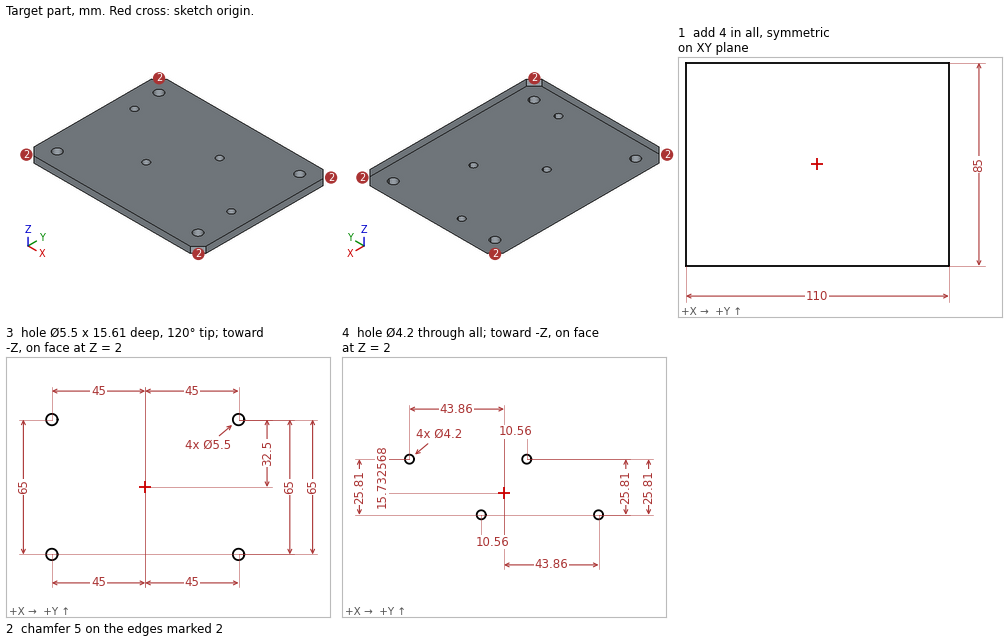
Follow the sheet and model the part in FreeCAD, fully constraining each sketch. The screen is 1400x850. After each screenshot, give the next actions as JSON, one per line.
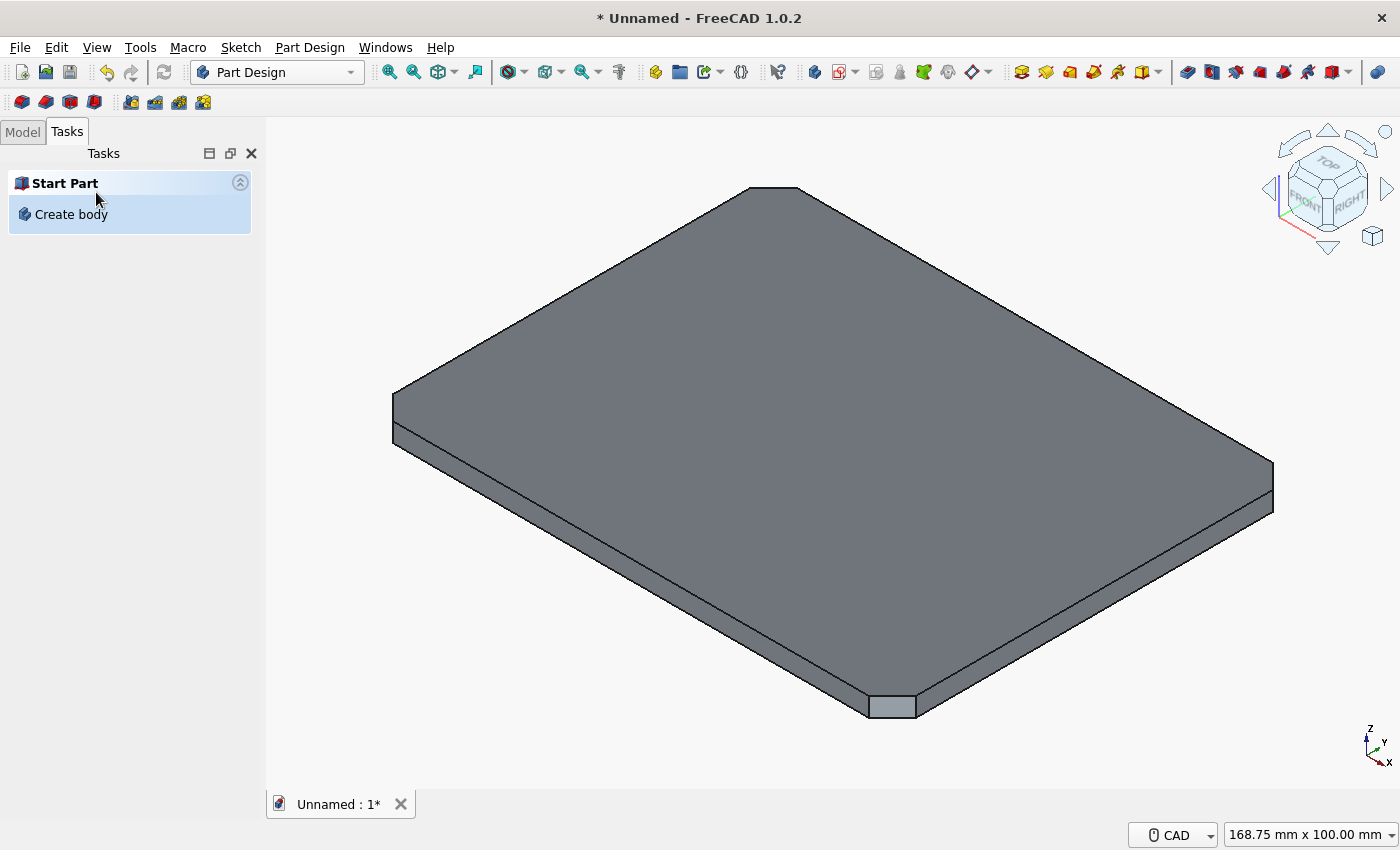
{"action": "left_click", "coordinate": [833, 441]}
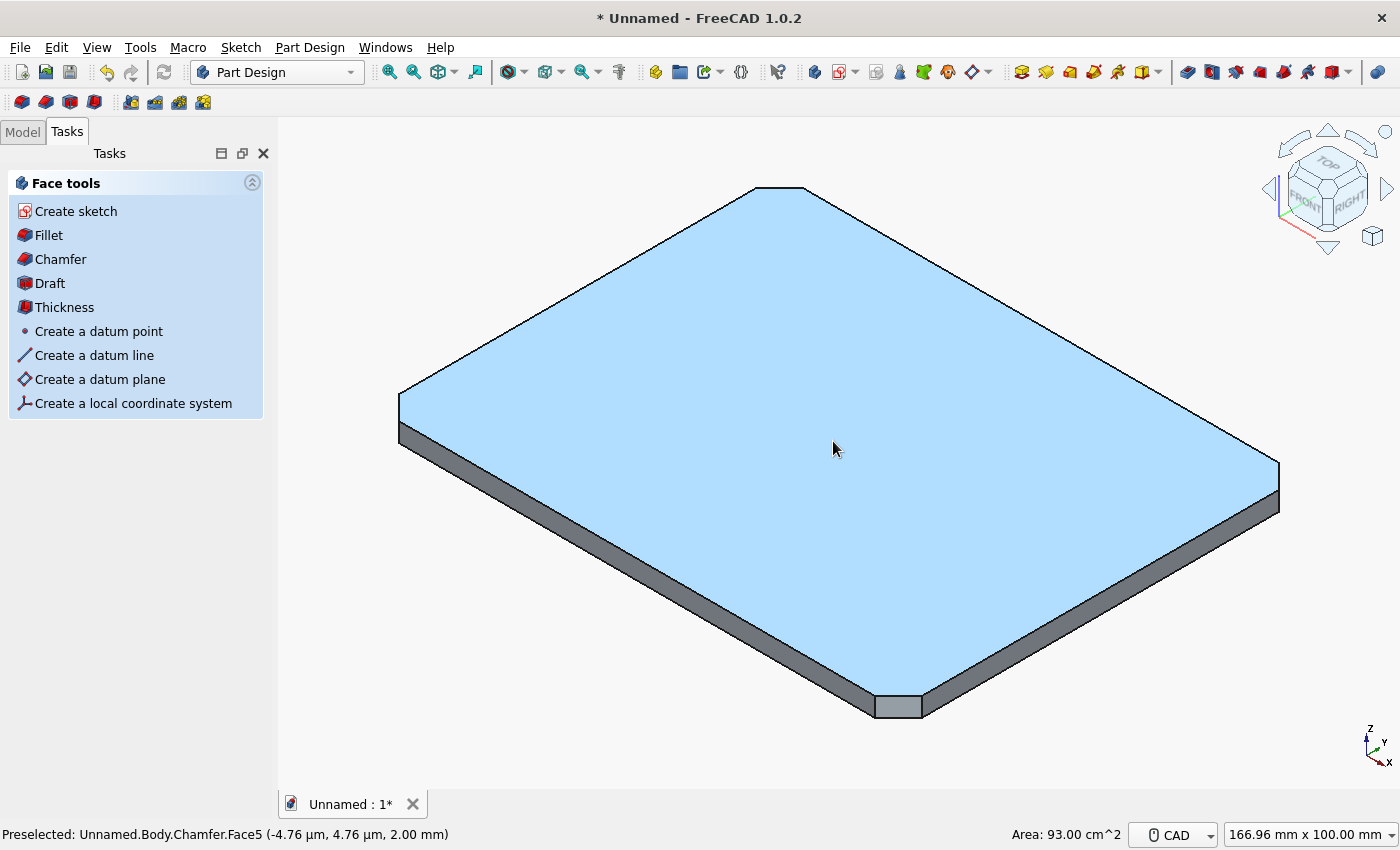
{"action": "left_click", "coordinate": [840, 72]}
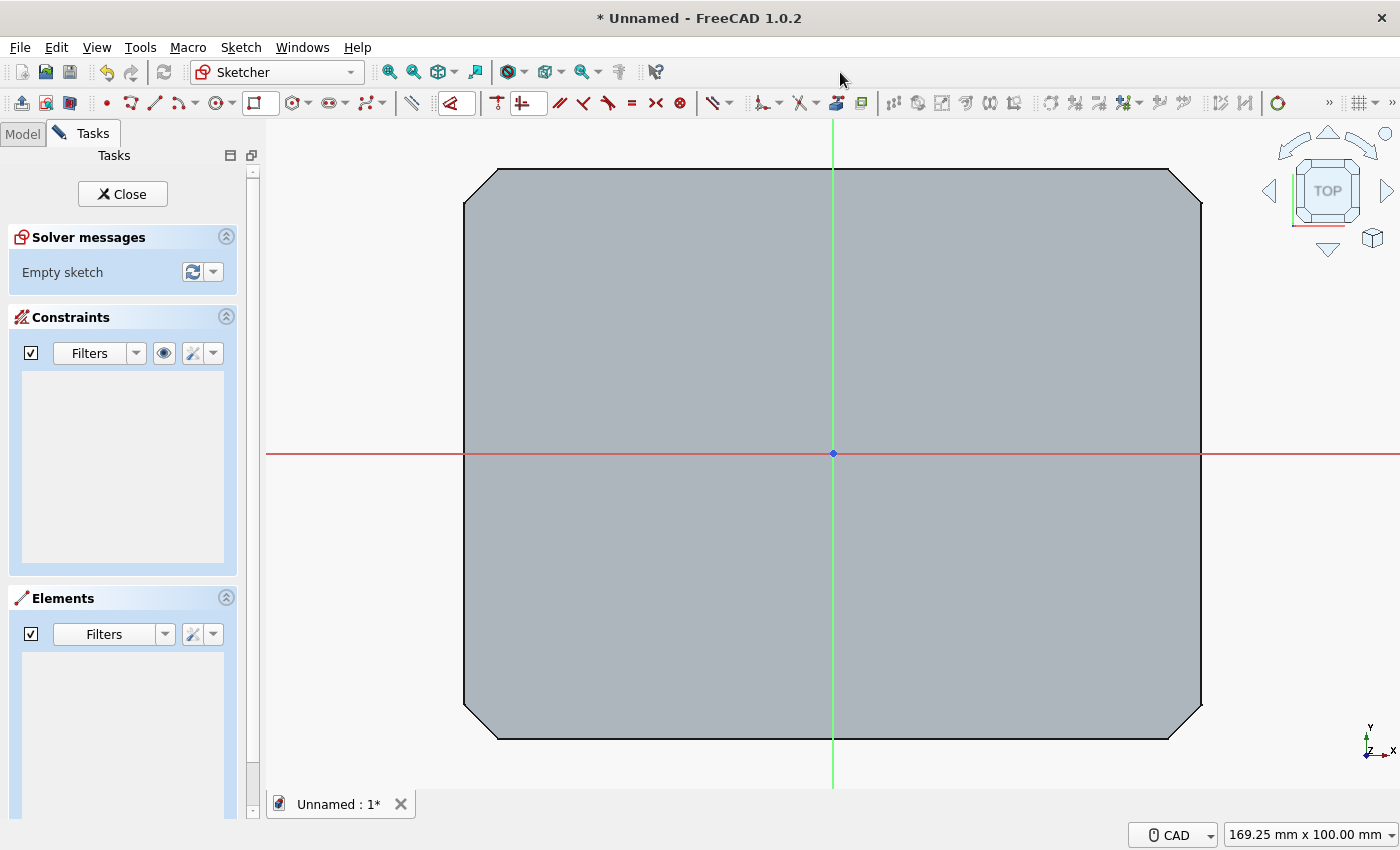
{"action": "left_click", "coordinate": [216, 104]}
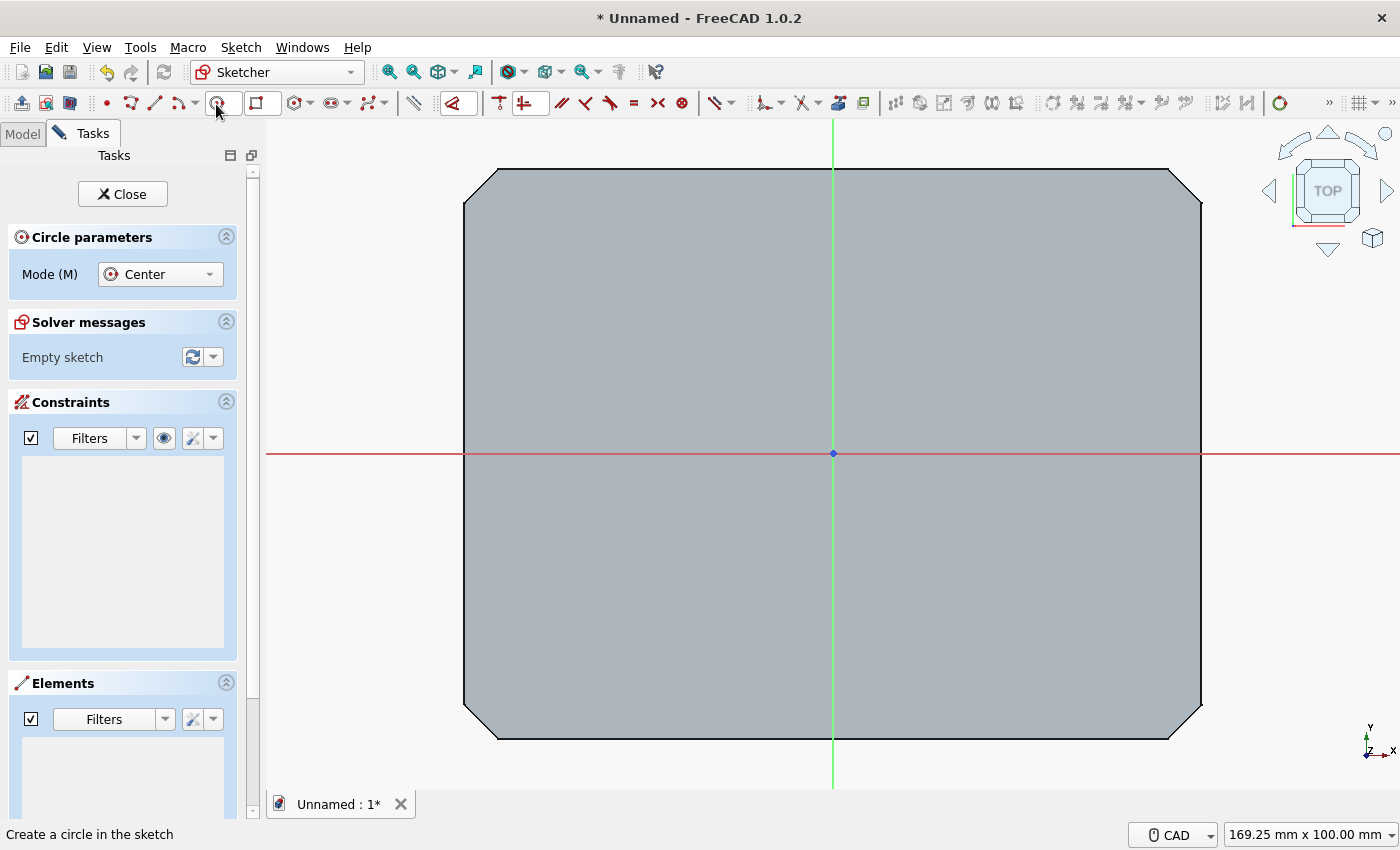
{"action": "scroll", "coordinate": [1134, 236], "scroll_direction": "up", "scroll_amount": 2}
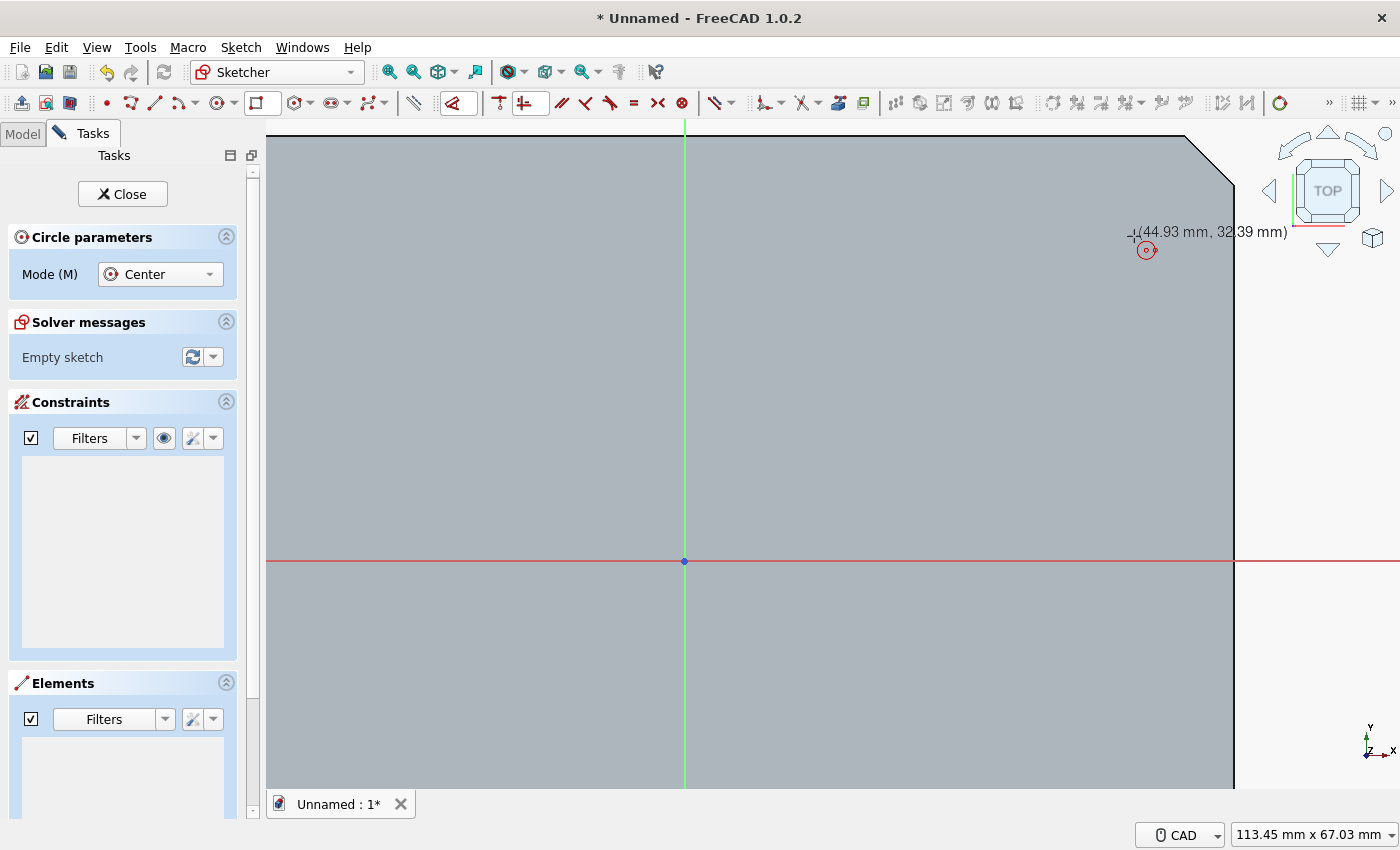
{"action": "left_click", "coordinate": [1134, 236]}
{"action": "mouse_move", "coordinate": [1154, 217]}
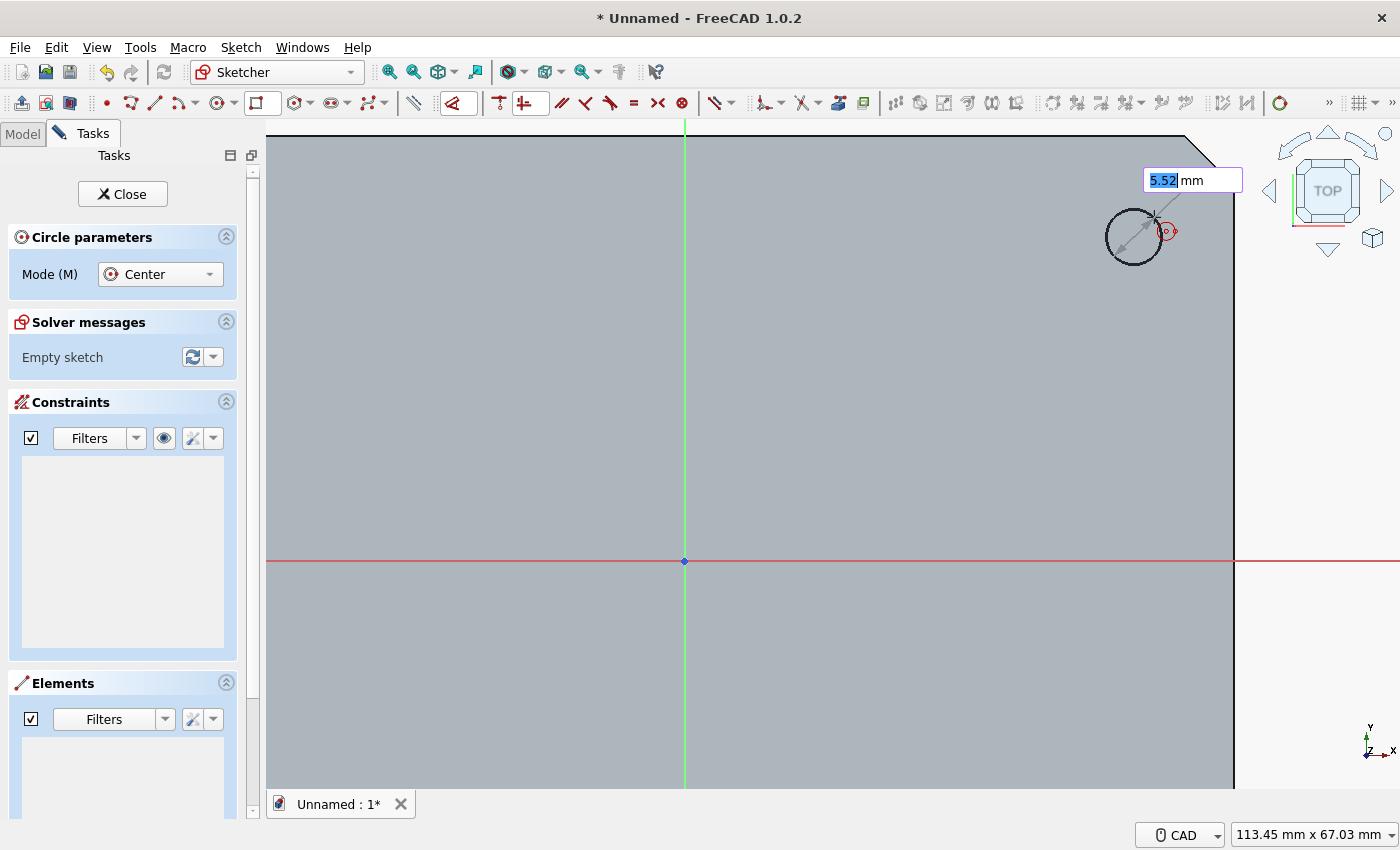
{"action": "type", "text": "5.5"}
{"action": "key", "text": "Return"}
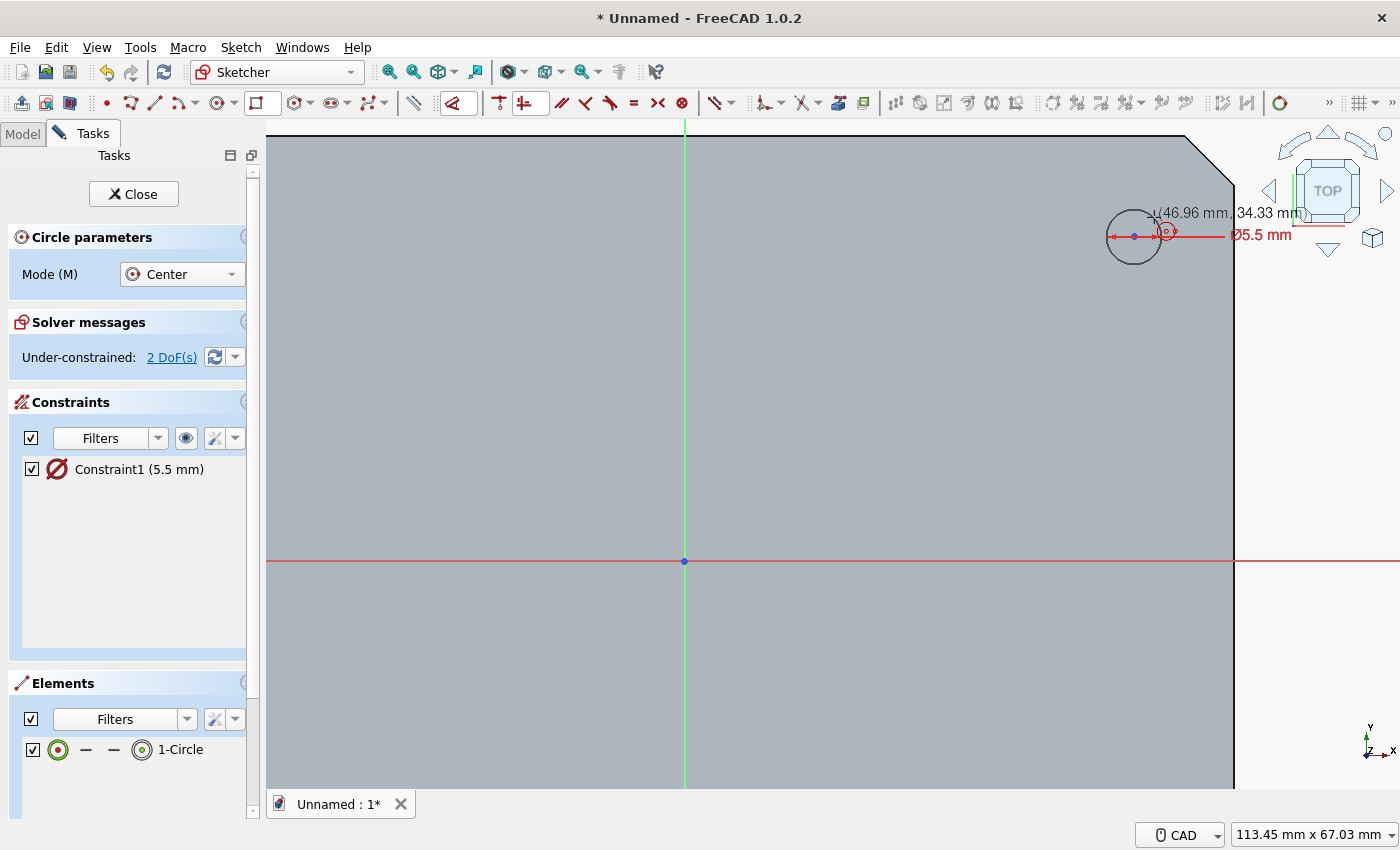
{"action": "scroll", "coordinate": [927, 236], "scroll_direction": "down", "scroll_amount": 2}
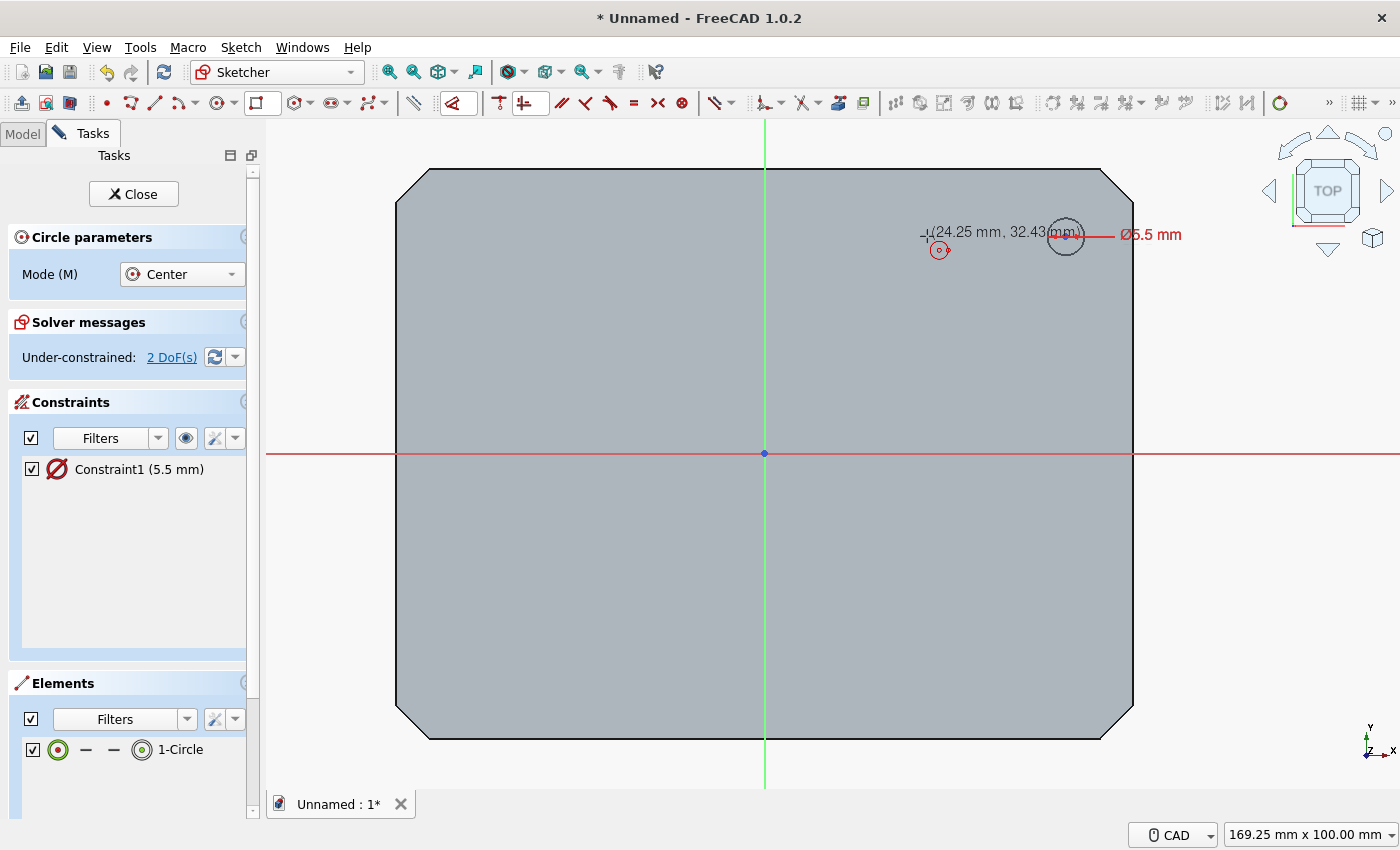
{"action": "scroll", "coordinate": [1066, 672], "scroll_direction": "up", "scroll_amount": 2}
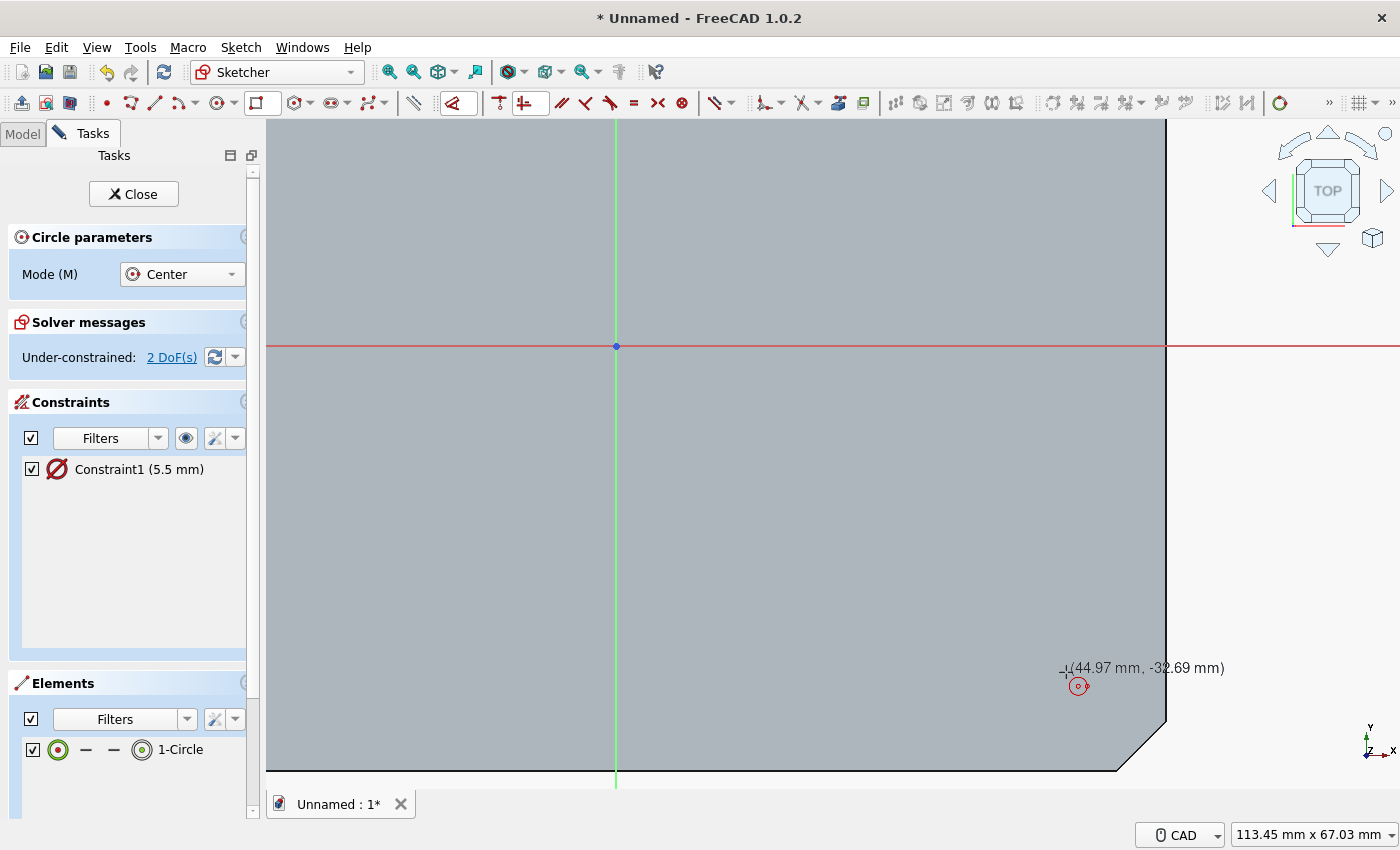
{"action": "left_click", "coordinate": [1066, 671]}
{"action": "mouse_move", "coordinate": [1085, 652]}